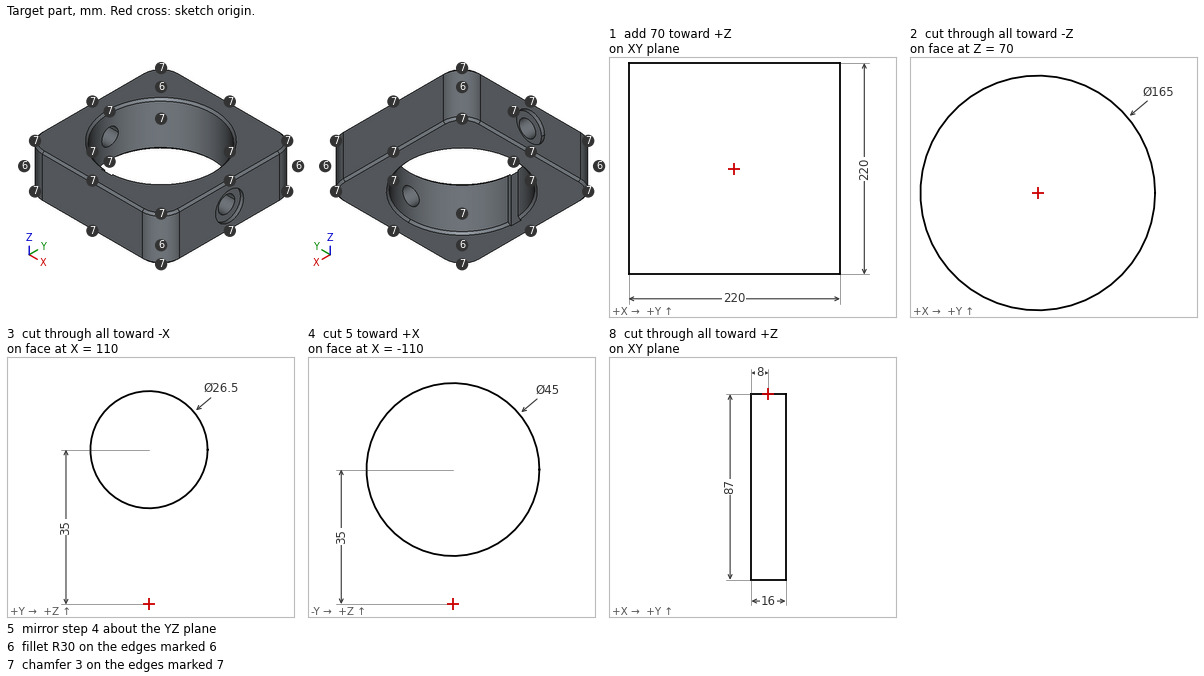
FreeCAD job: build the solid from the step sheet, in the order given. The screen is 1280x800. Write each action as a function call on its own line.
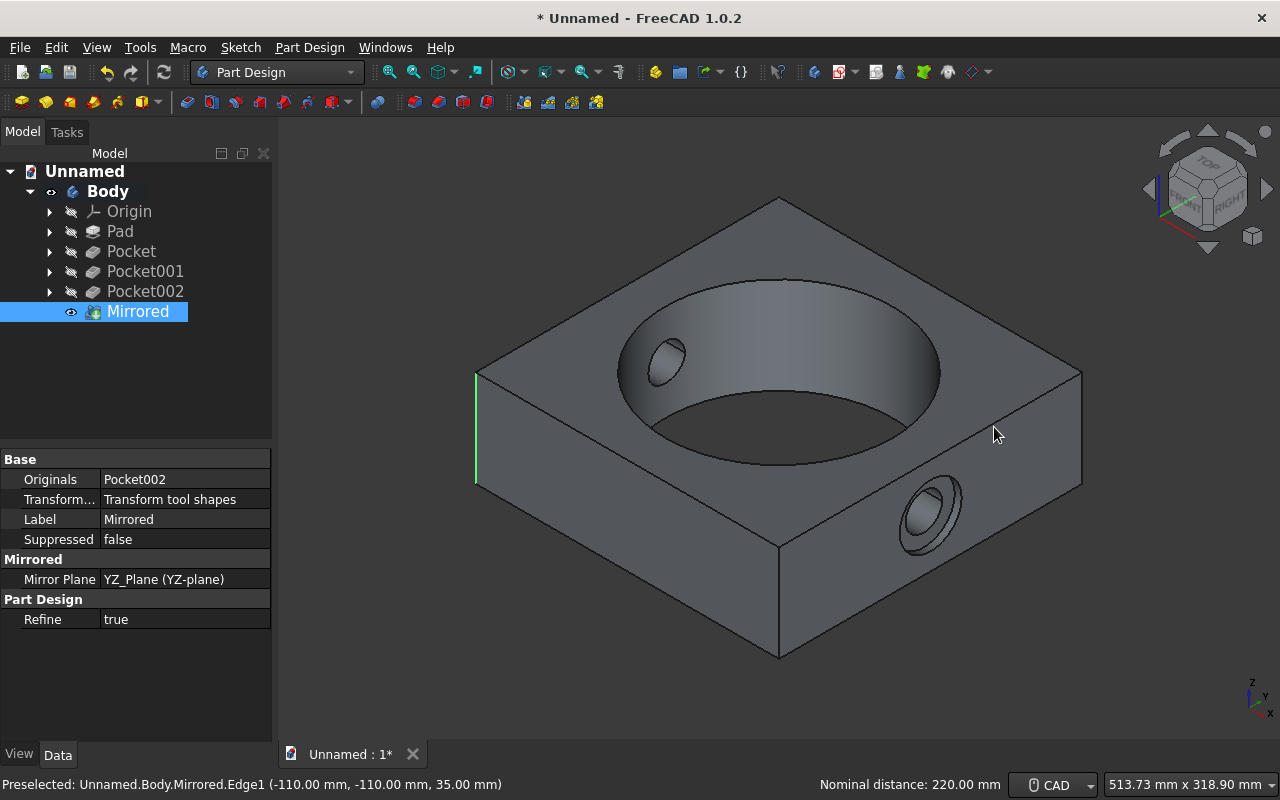
click(779, 602, ctrl)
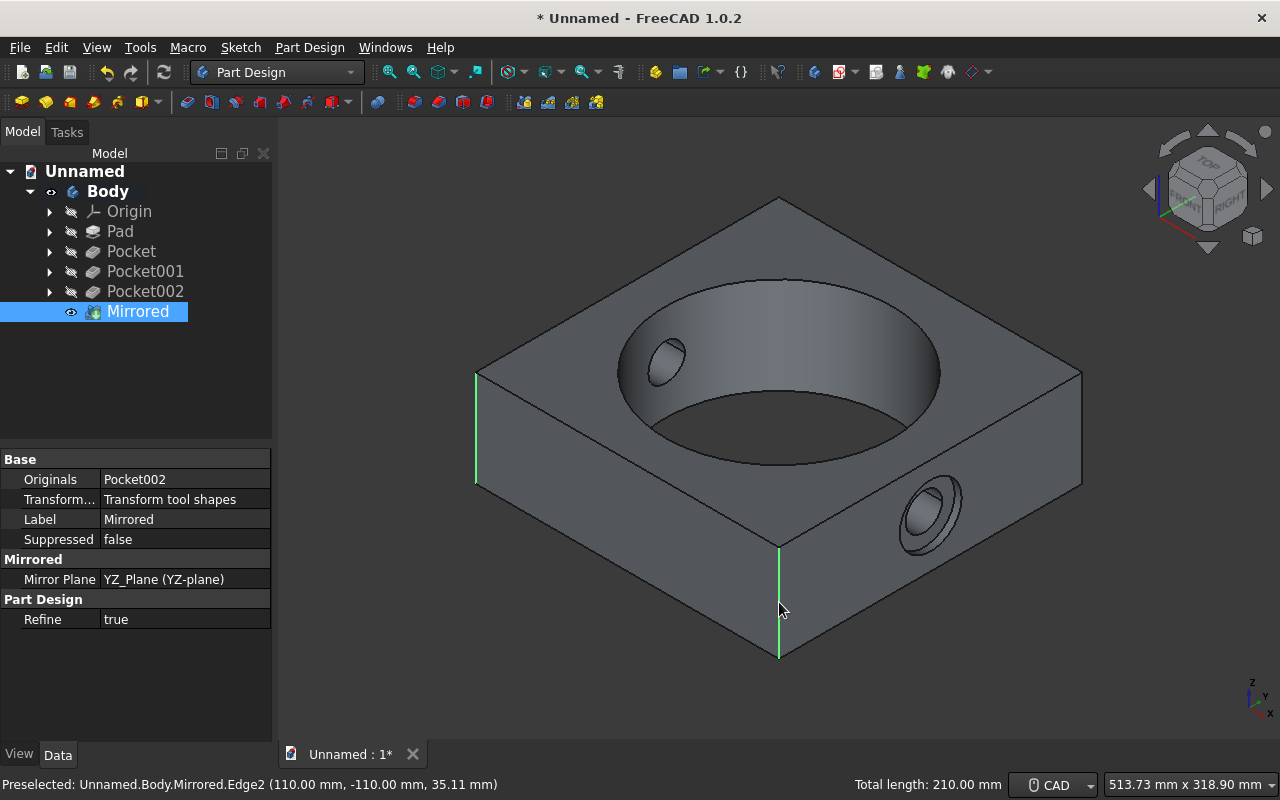
key(2)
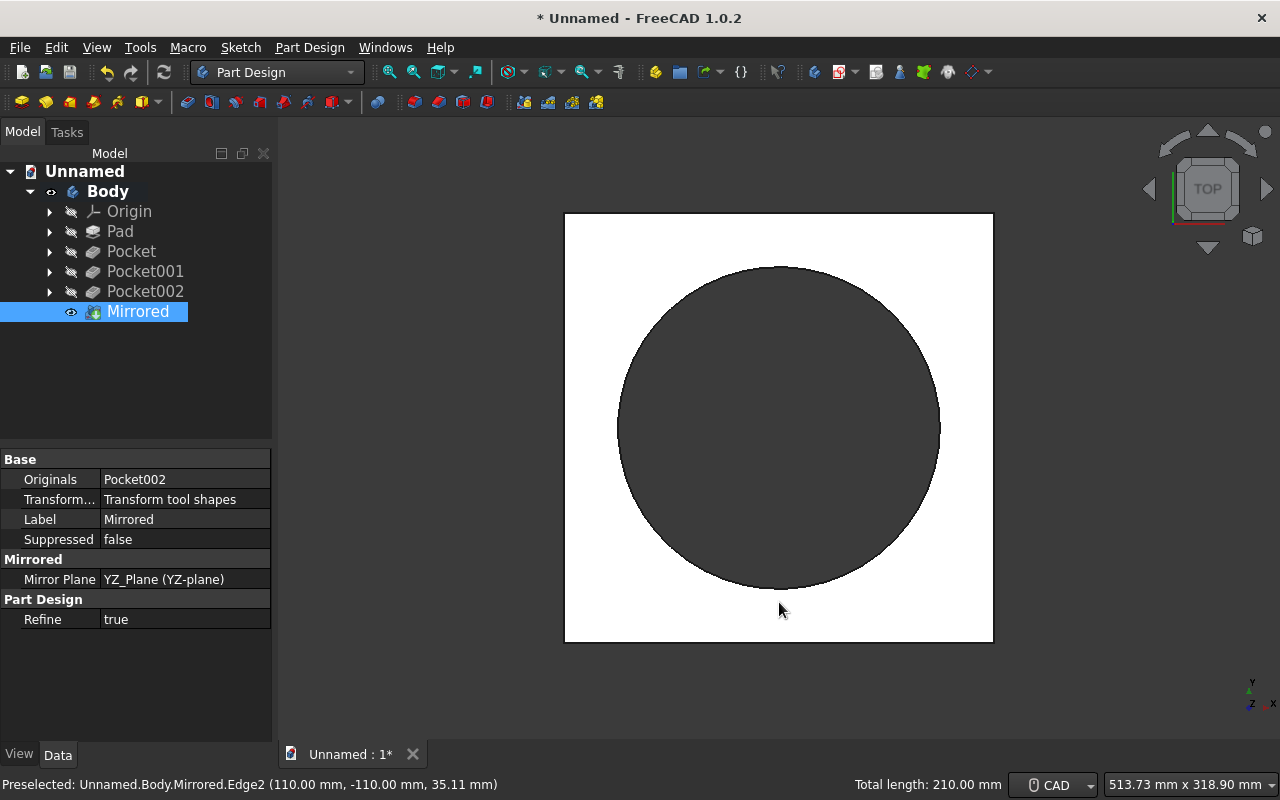
key(1)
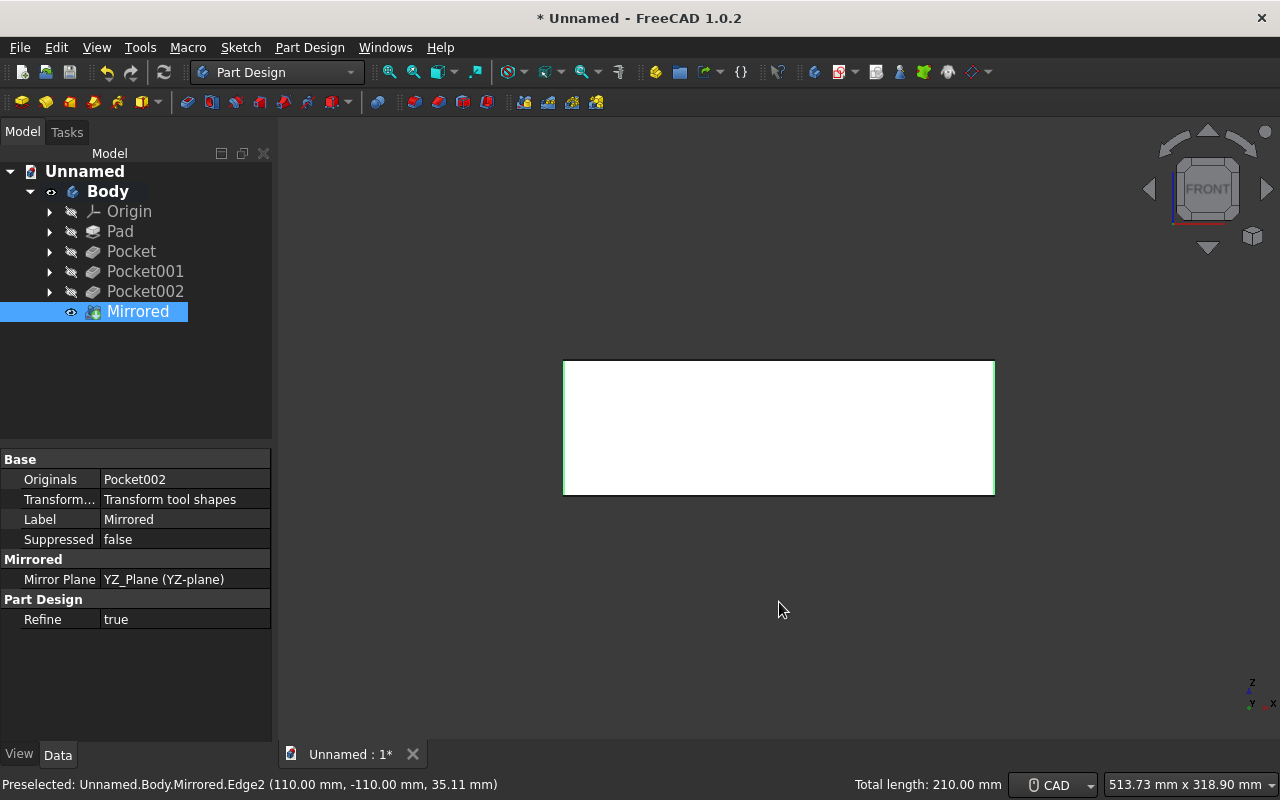
key(v)
key(f)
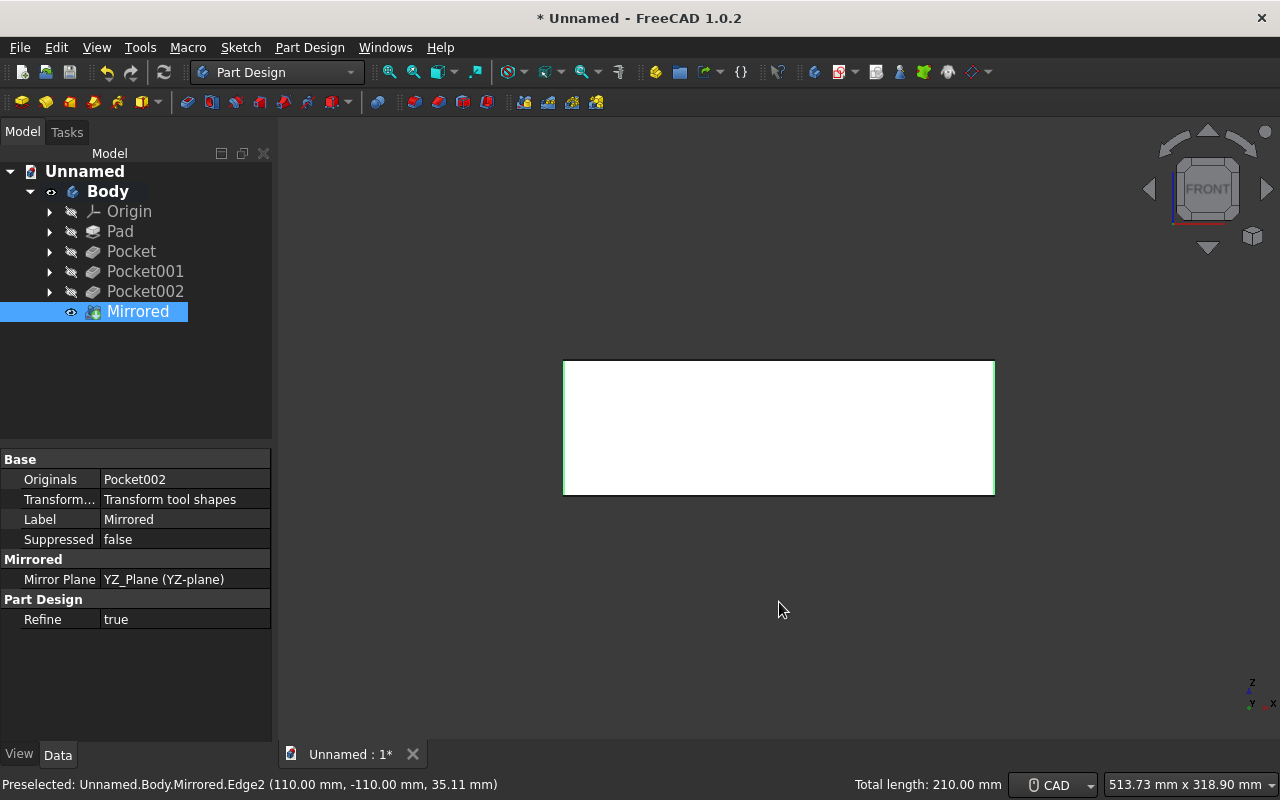
key(3)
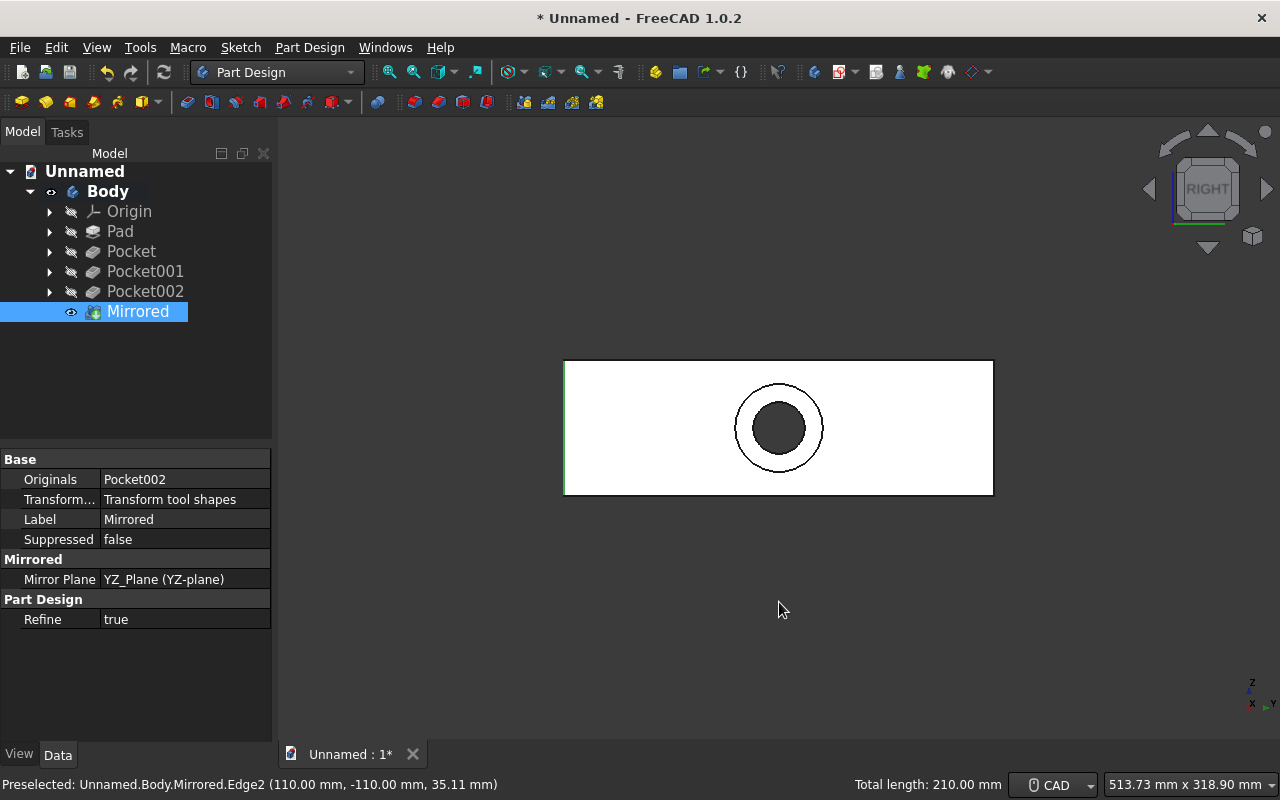
click(390, 72)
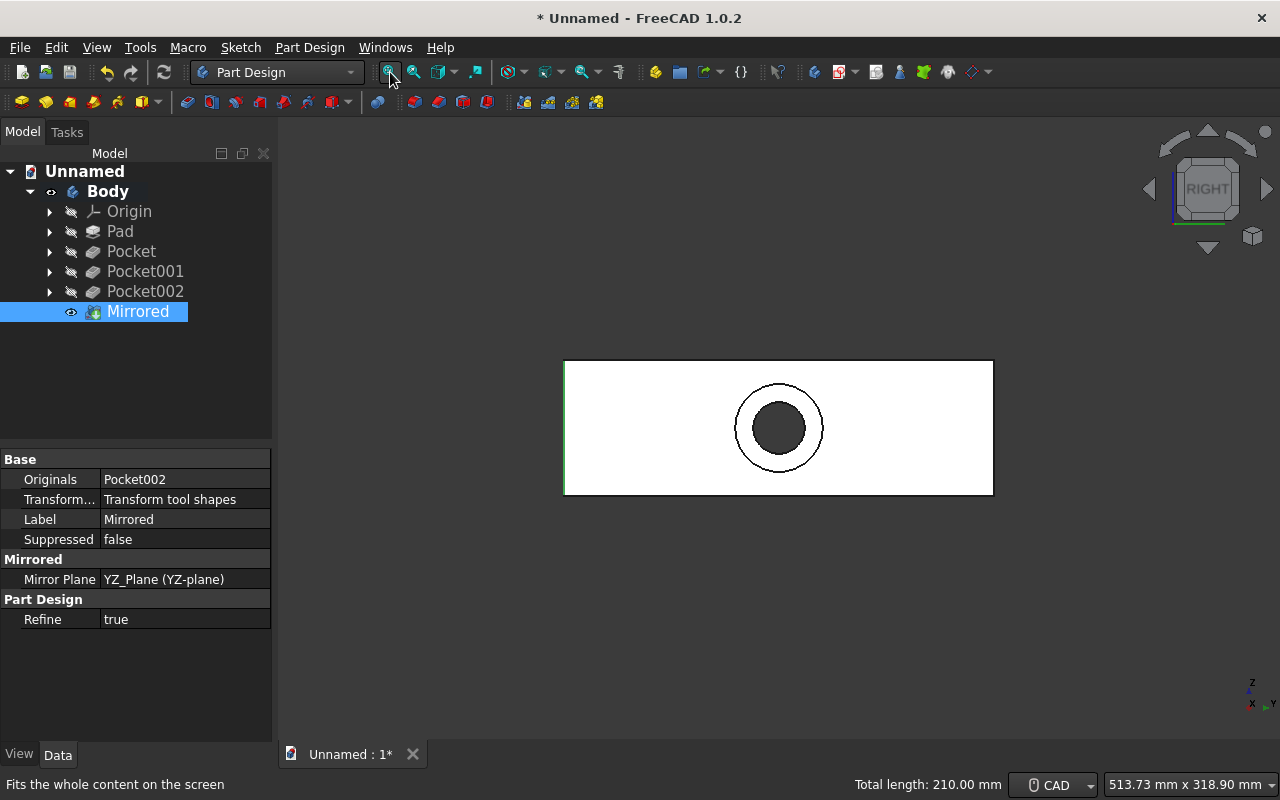
click(994, 427, ctrl)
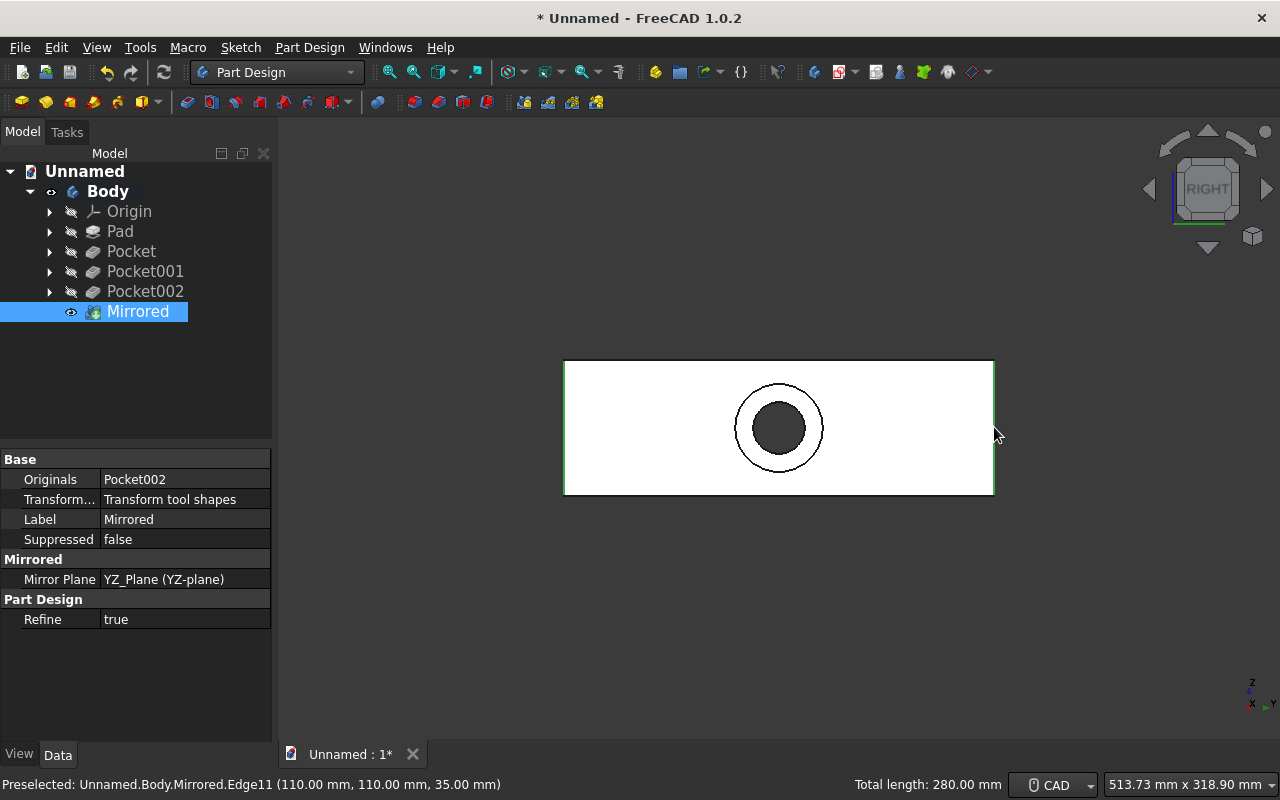
click(416, 102)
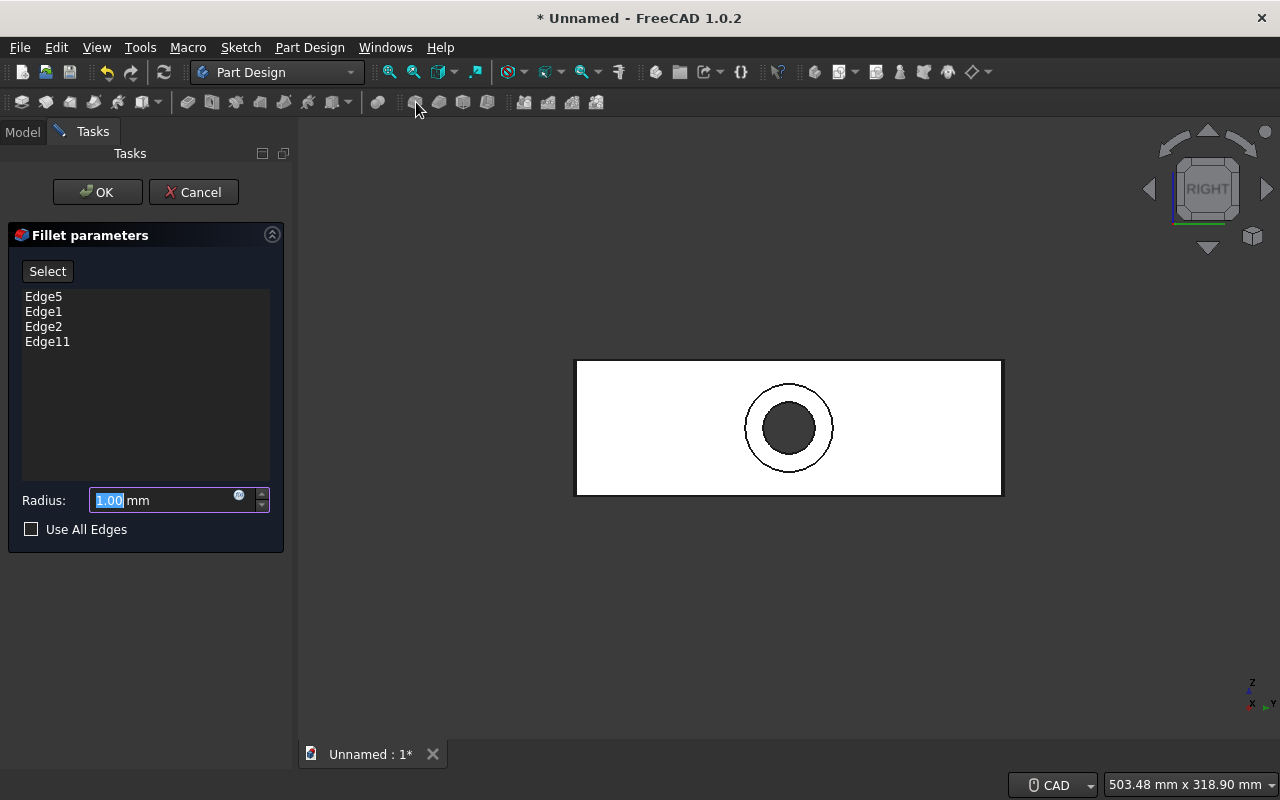
text(30)
key(Tab)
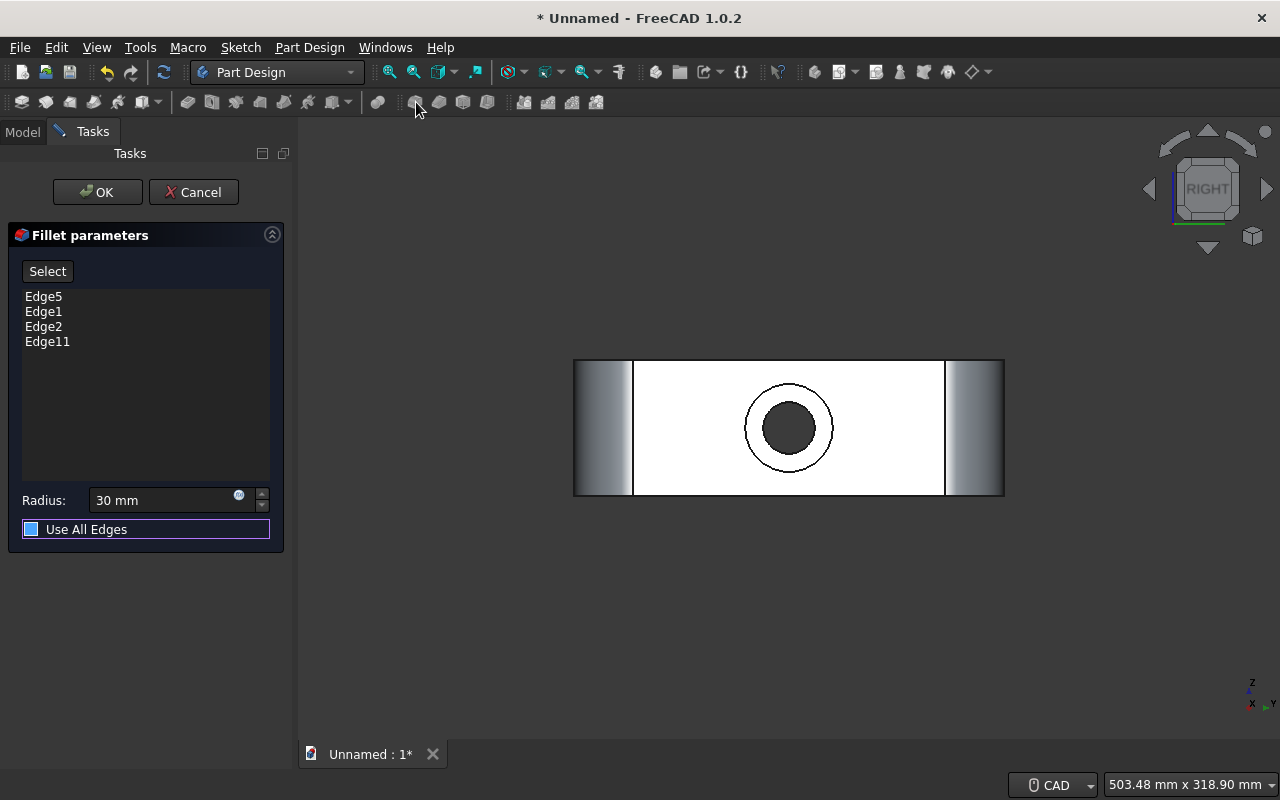
click(98, 192)